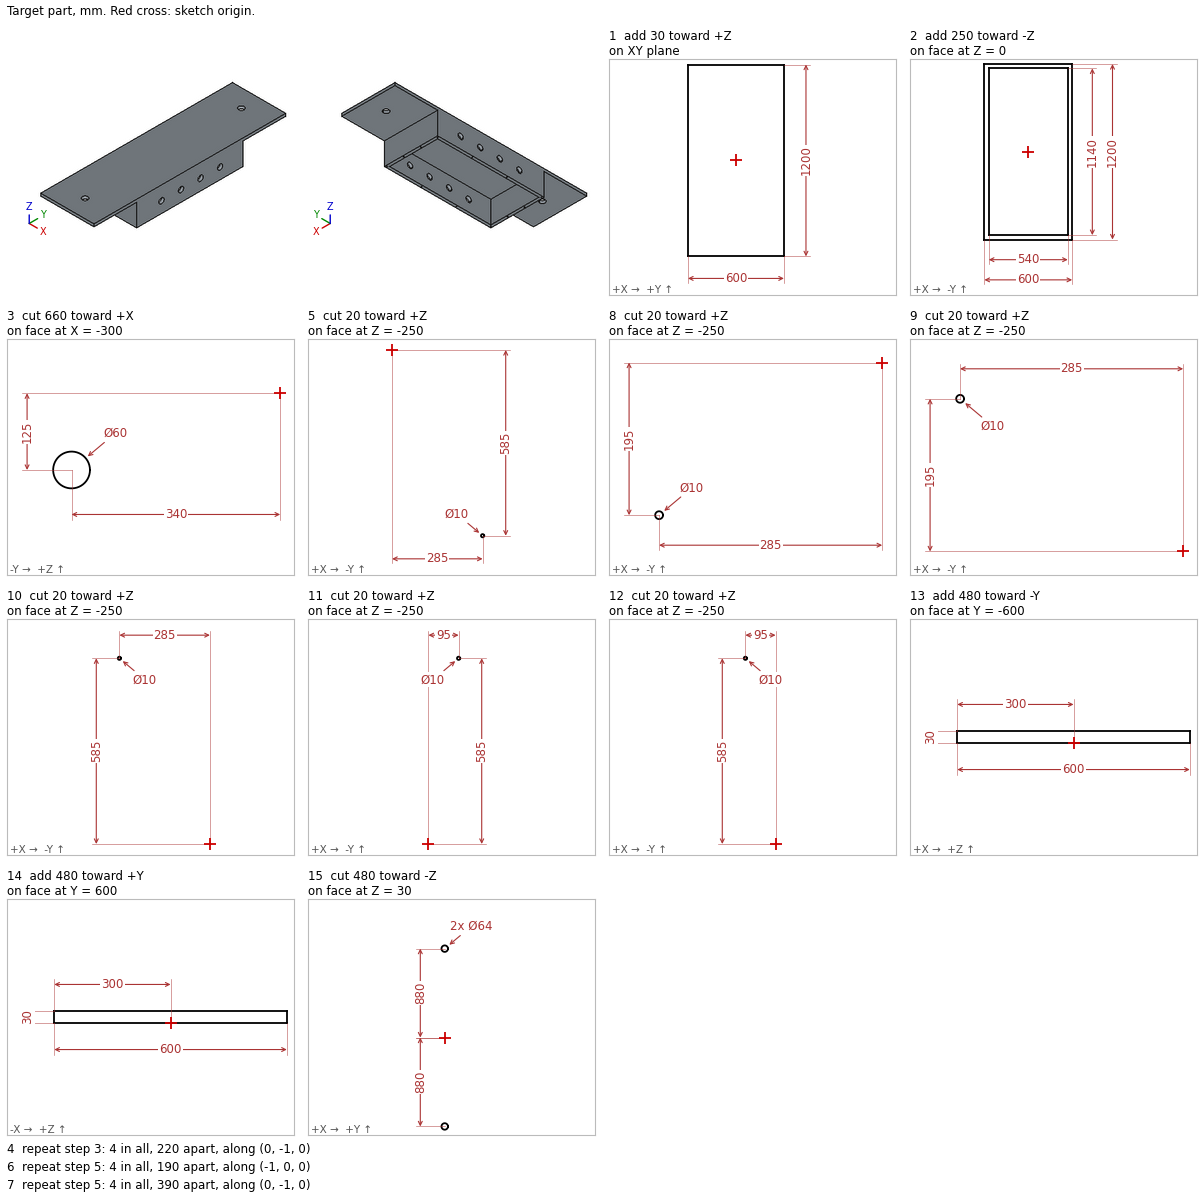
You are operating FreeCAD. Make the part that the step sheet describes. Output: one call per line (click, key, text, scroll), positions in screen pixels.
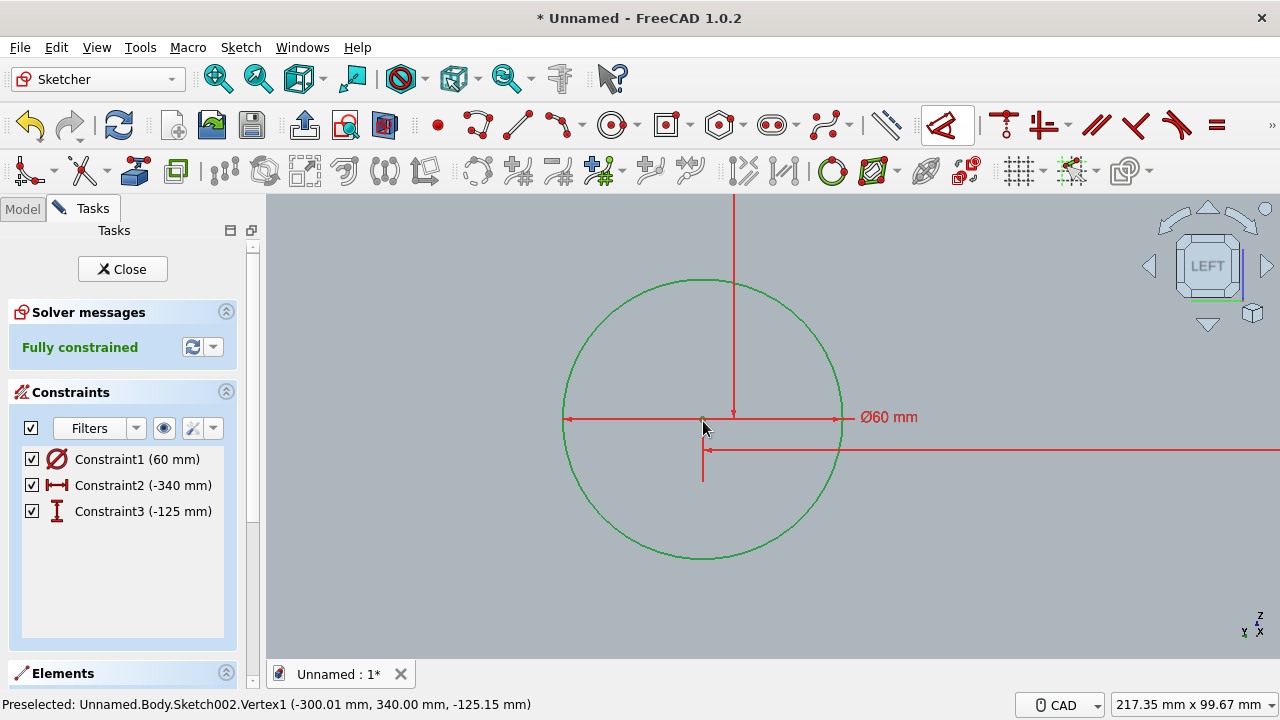
click(123, 269)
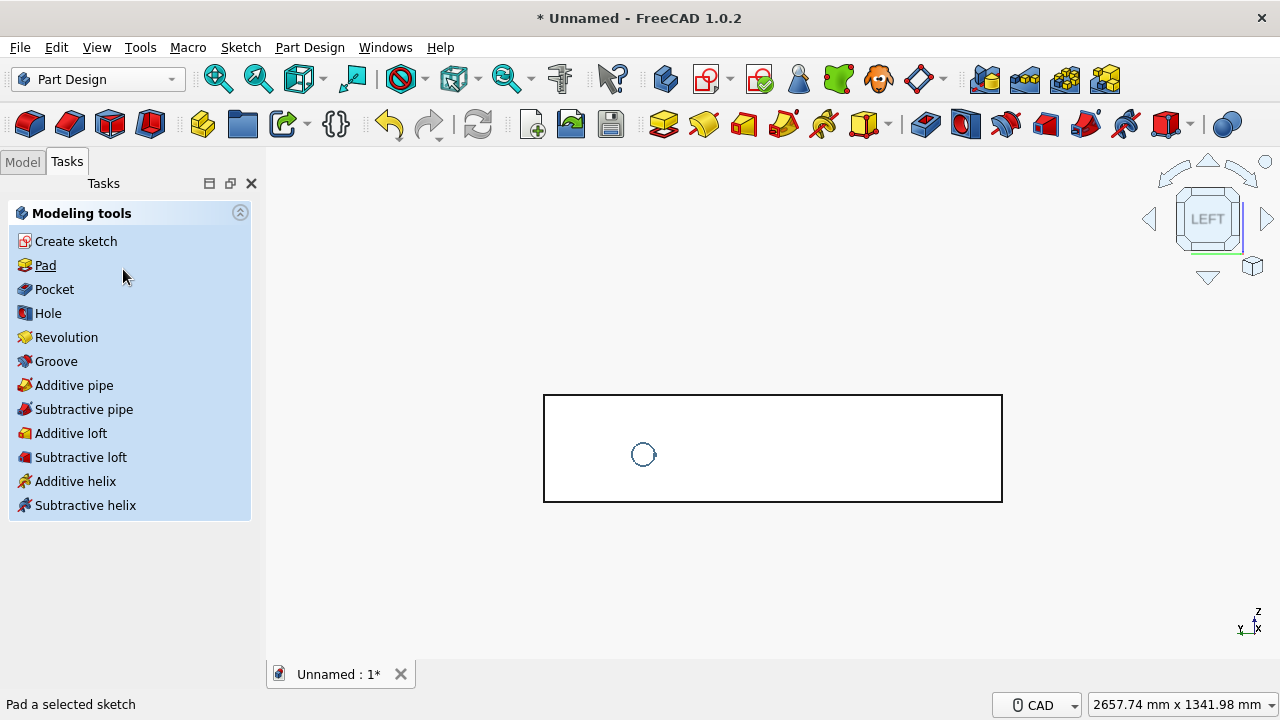
click(926, 124)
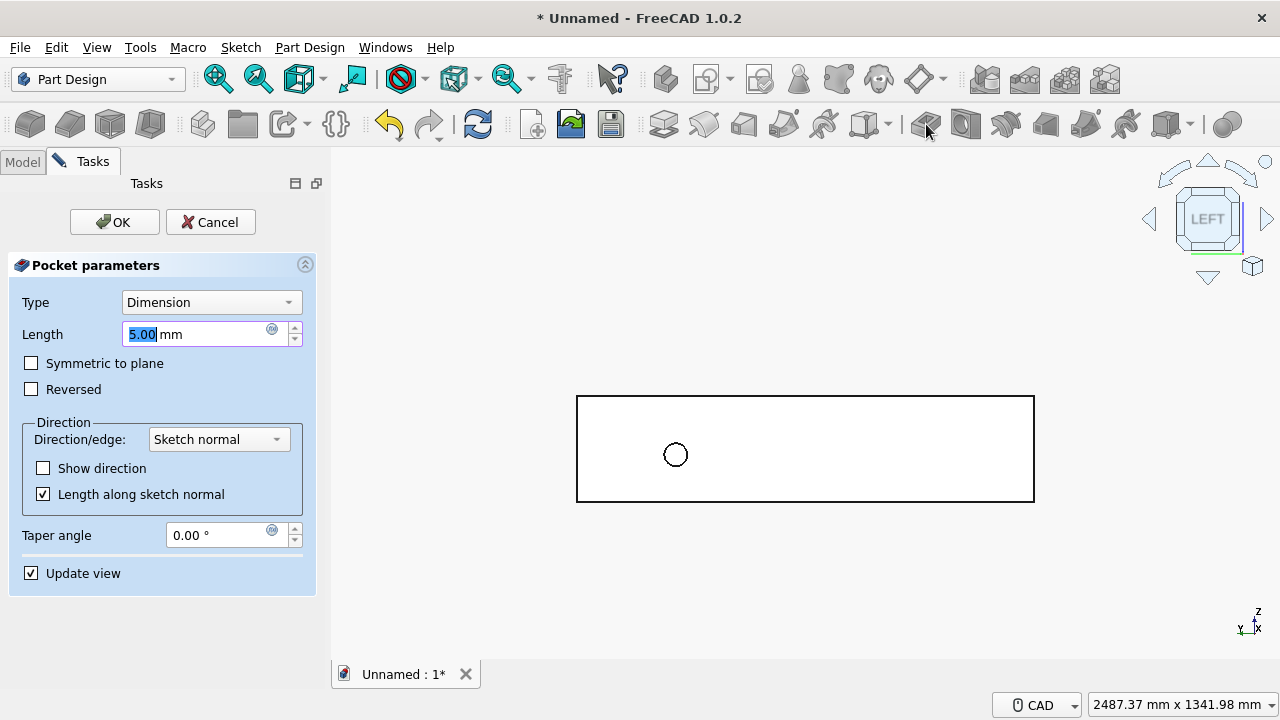
text(660)
key(Tab)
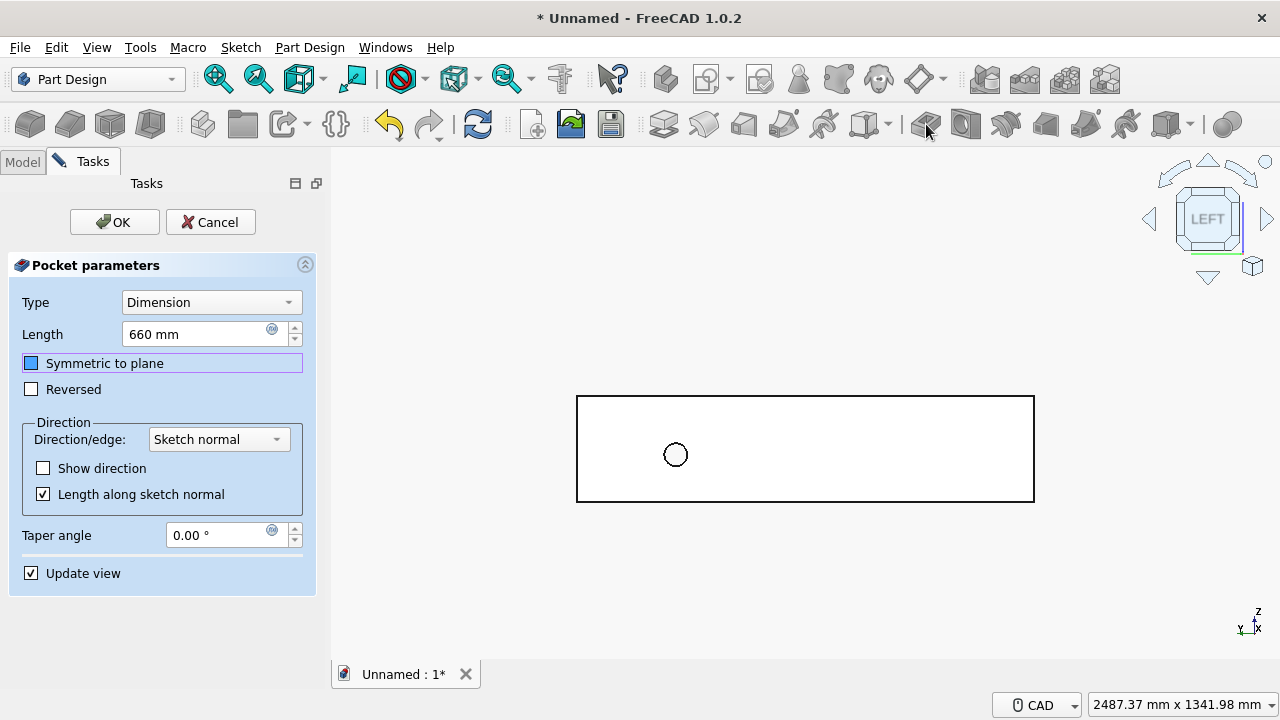
click(115, 222)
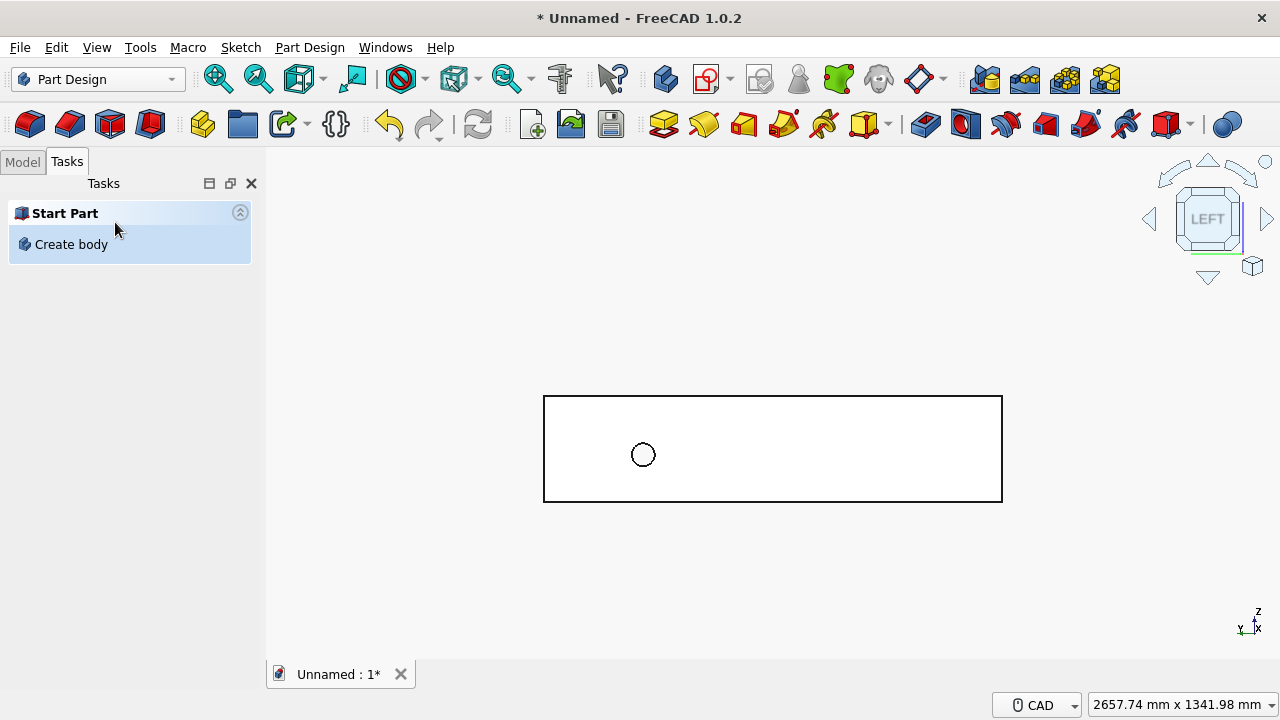
click(23, 161)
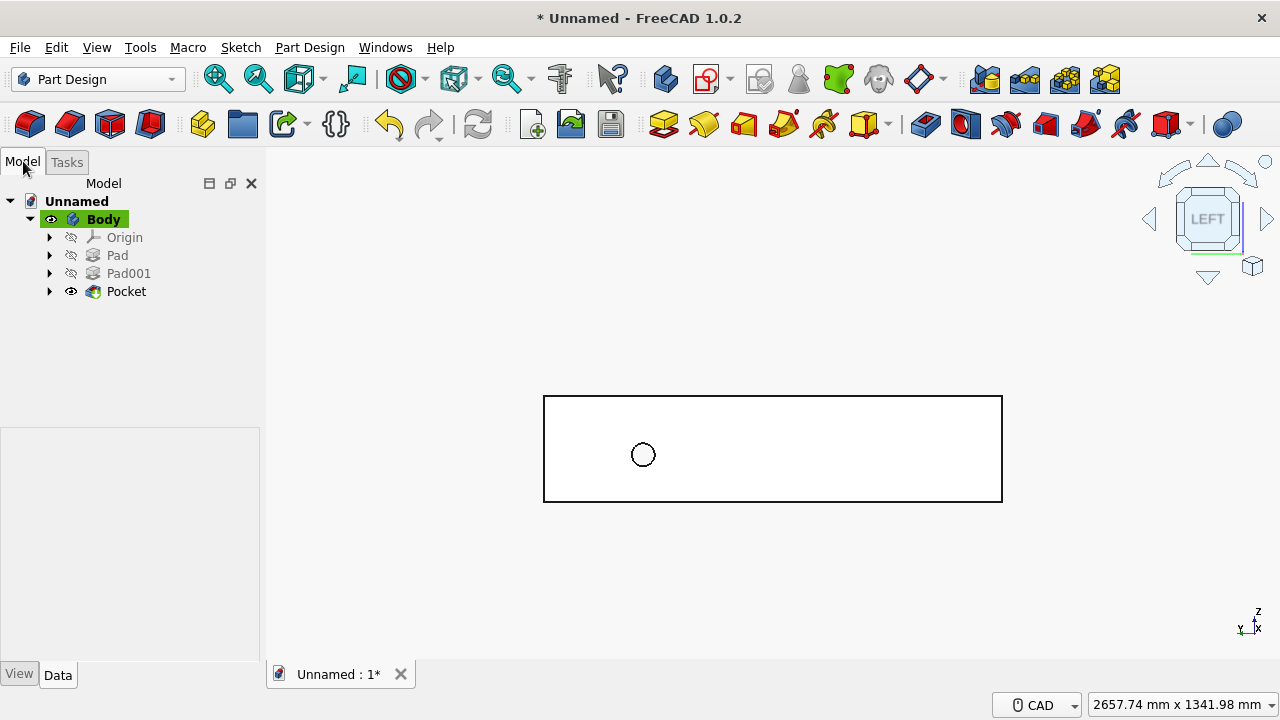
click(116, 291)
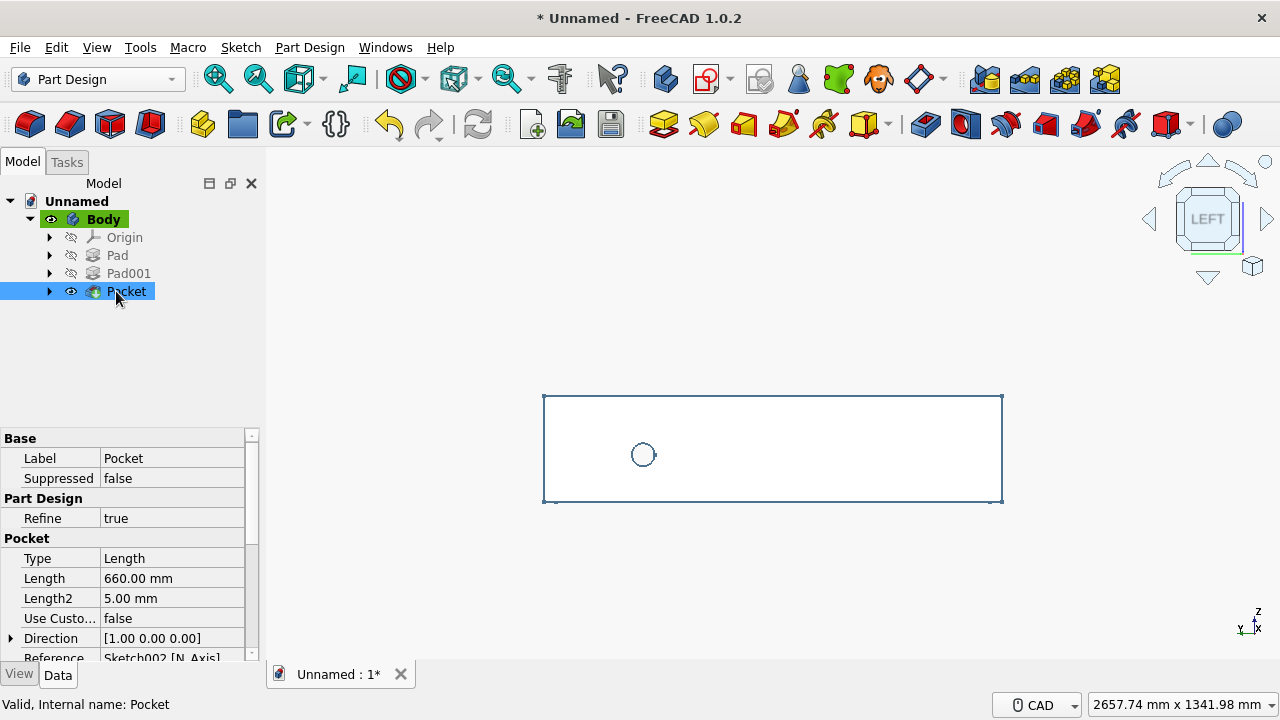
click(1026, 80)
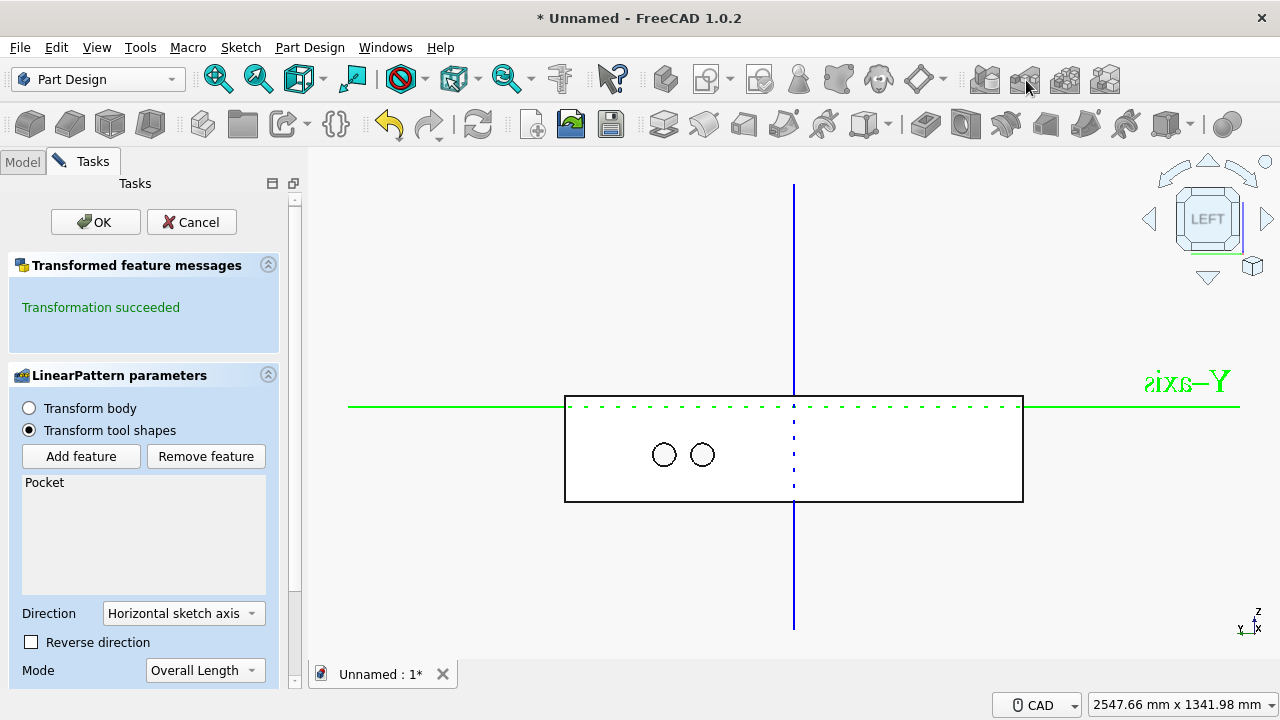
click(184, 614)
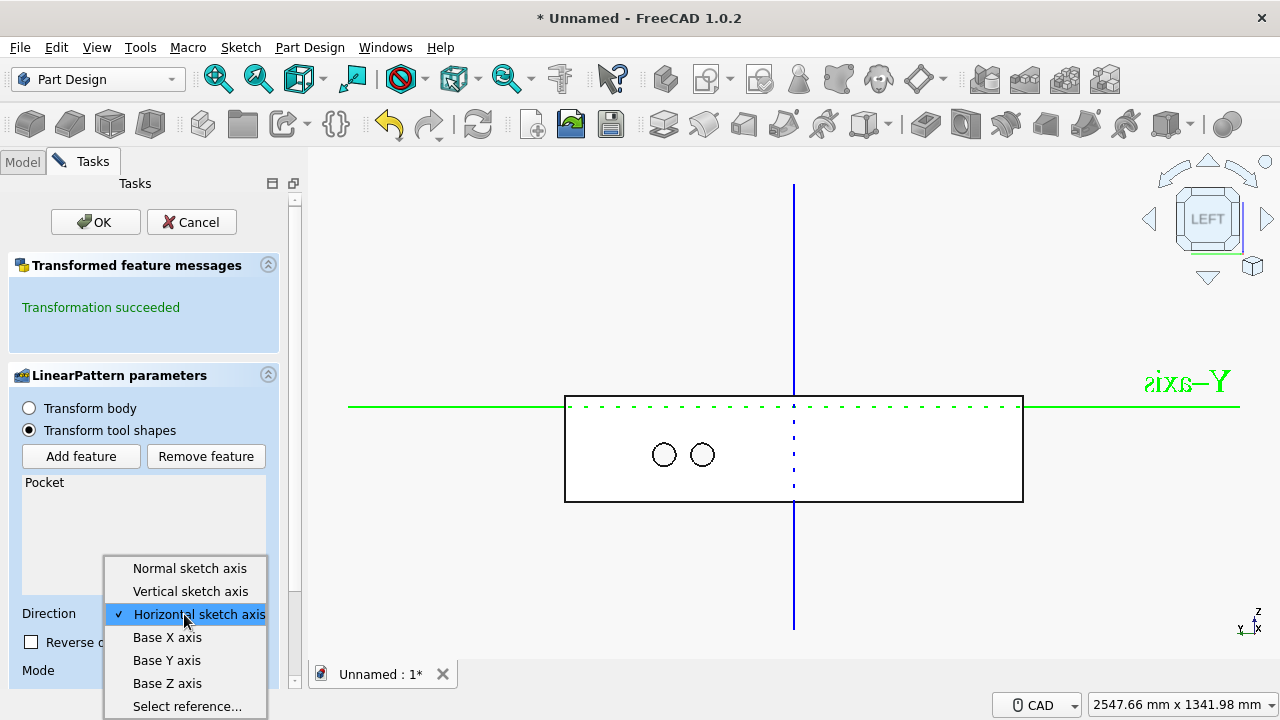
click(184, 660)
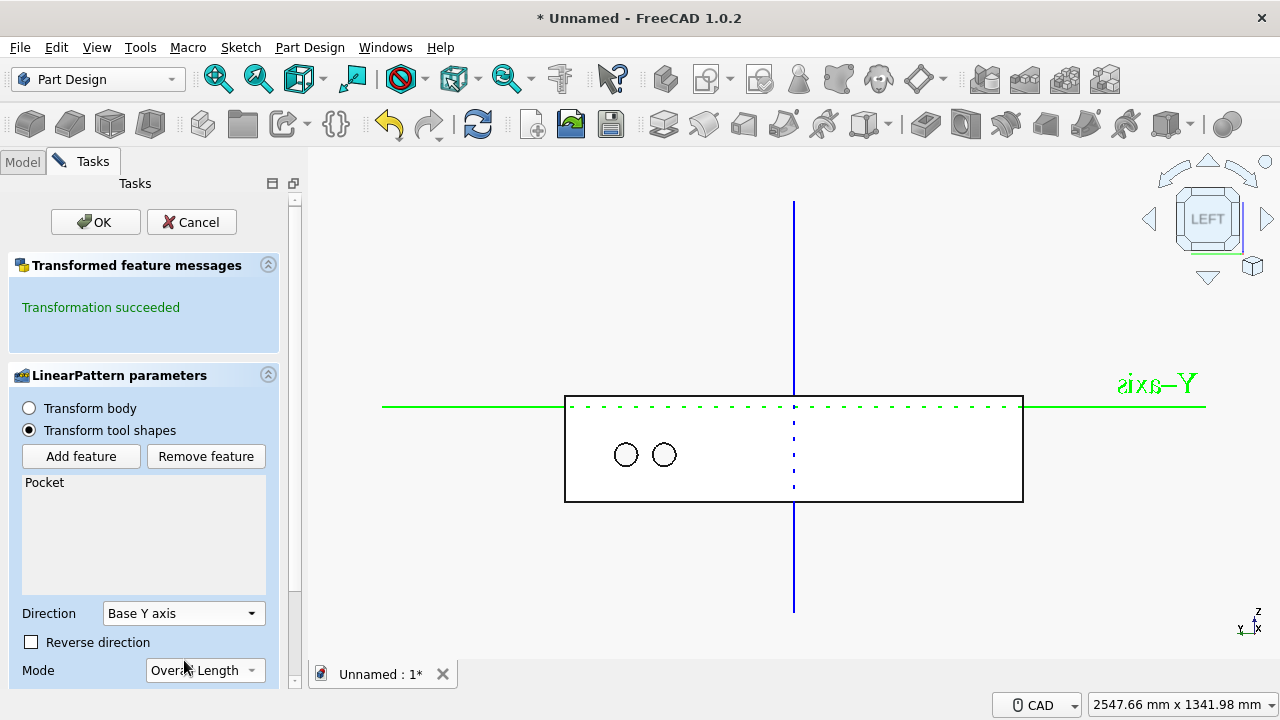
click(206, 670)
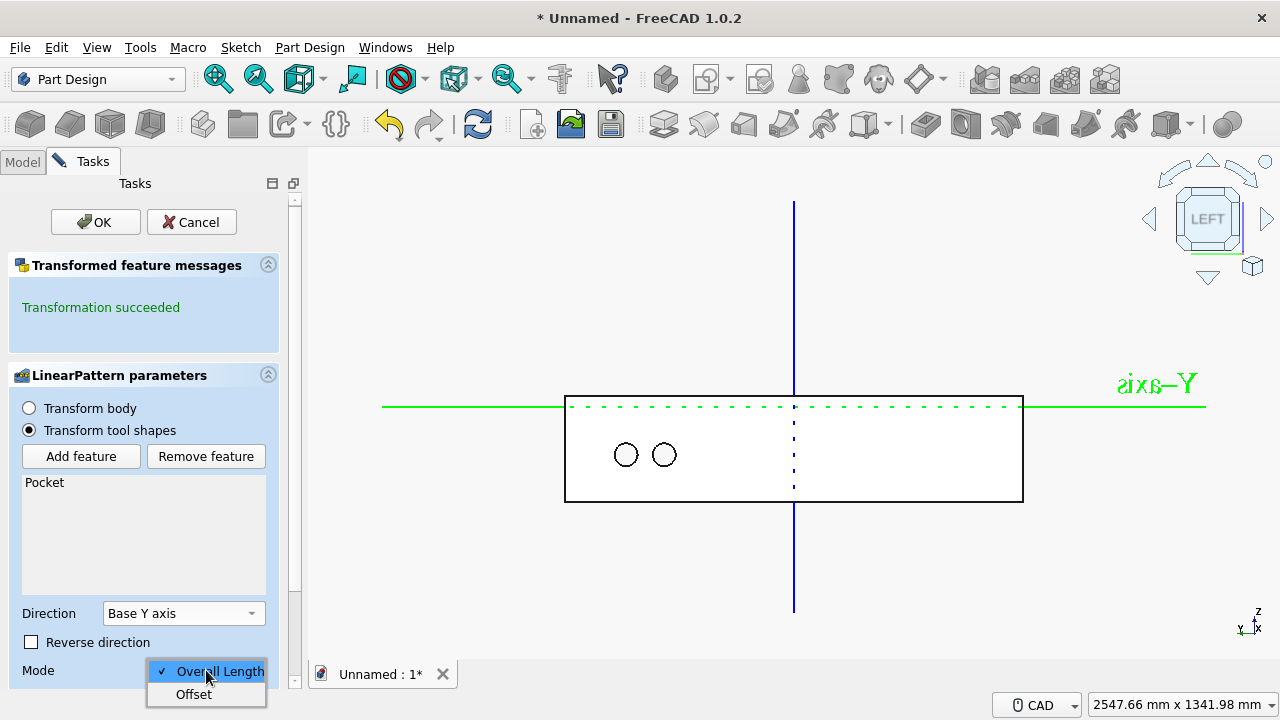
click(206, 694)